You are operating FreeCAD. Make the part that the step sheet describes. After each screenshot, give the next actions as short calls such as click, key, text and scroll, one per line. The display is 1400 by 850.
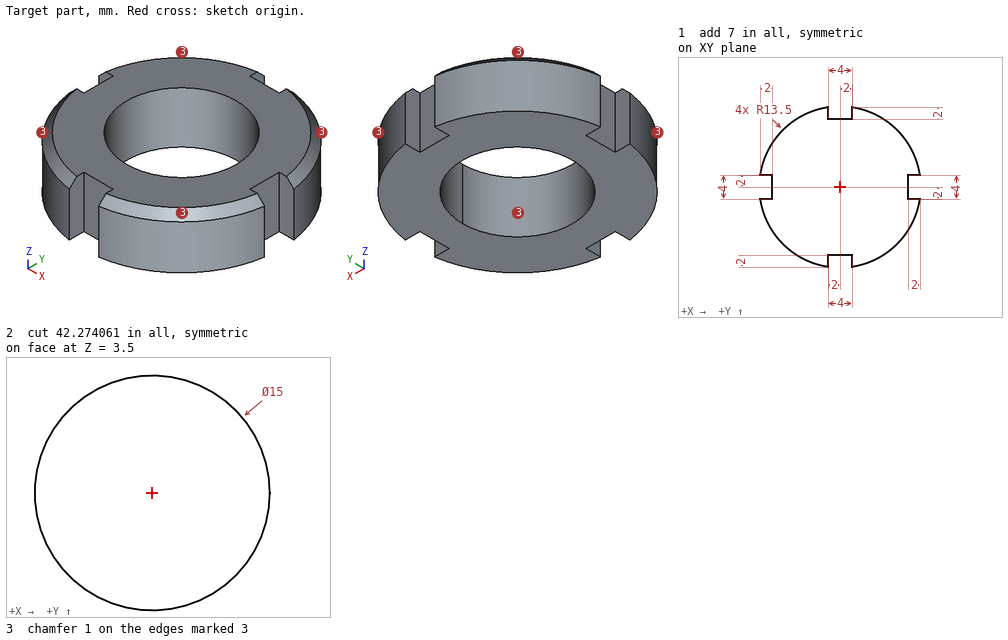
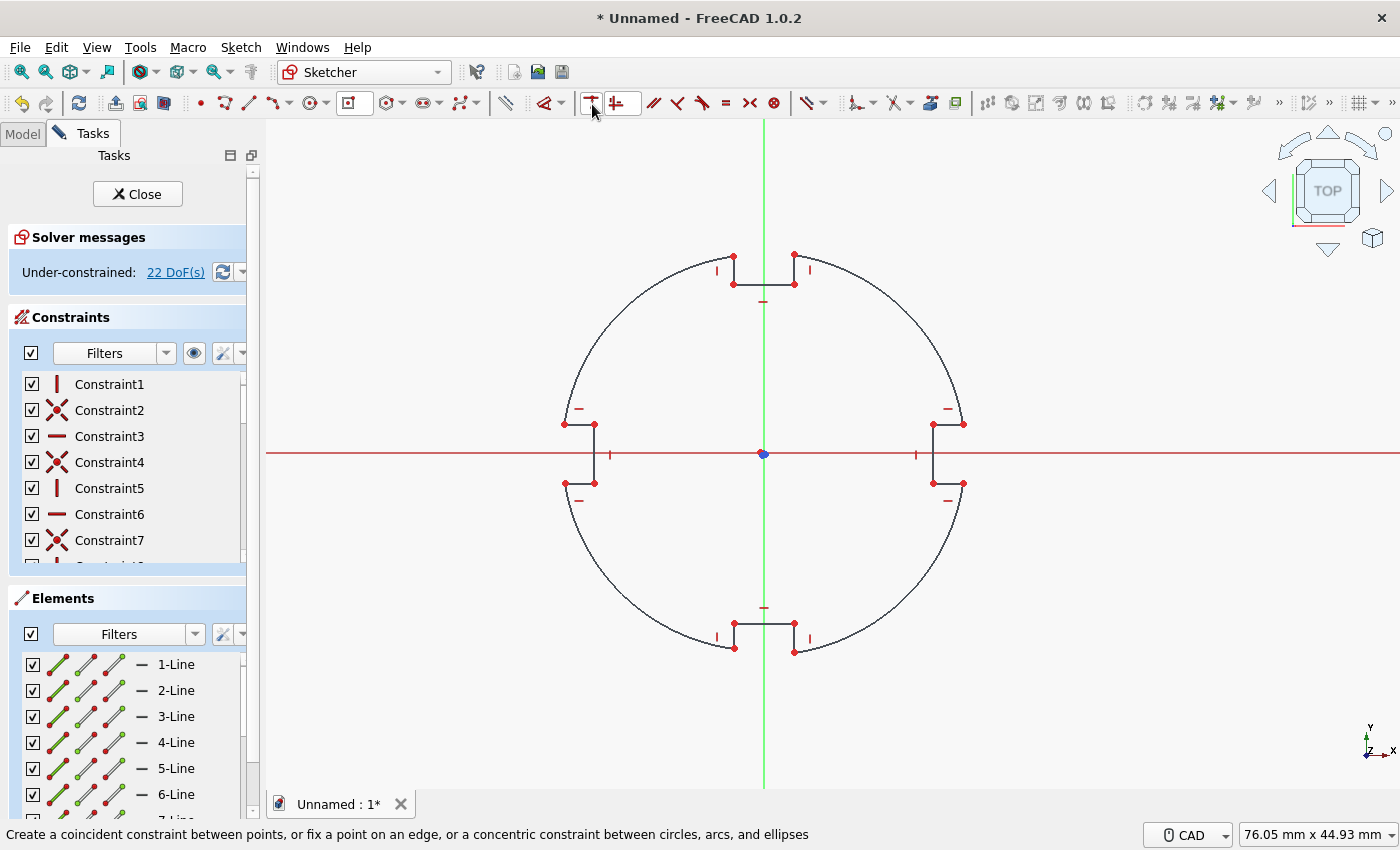
click(662, 281)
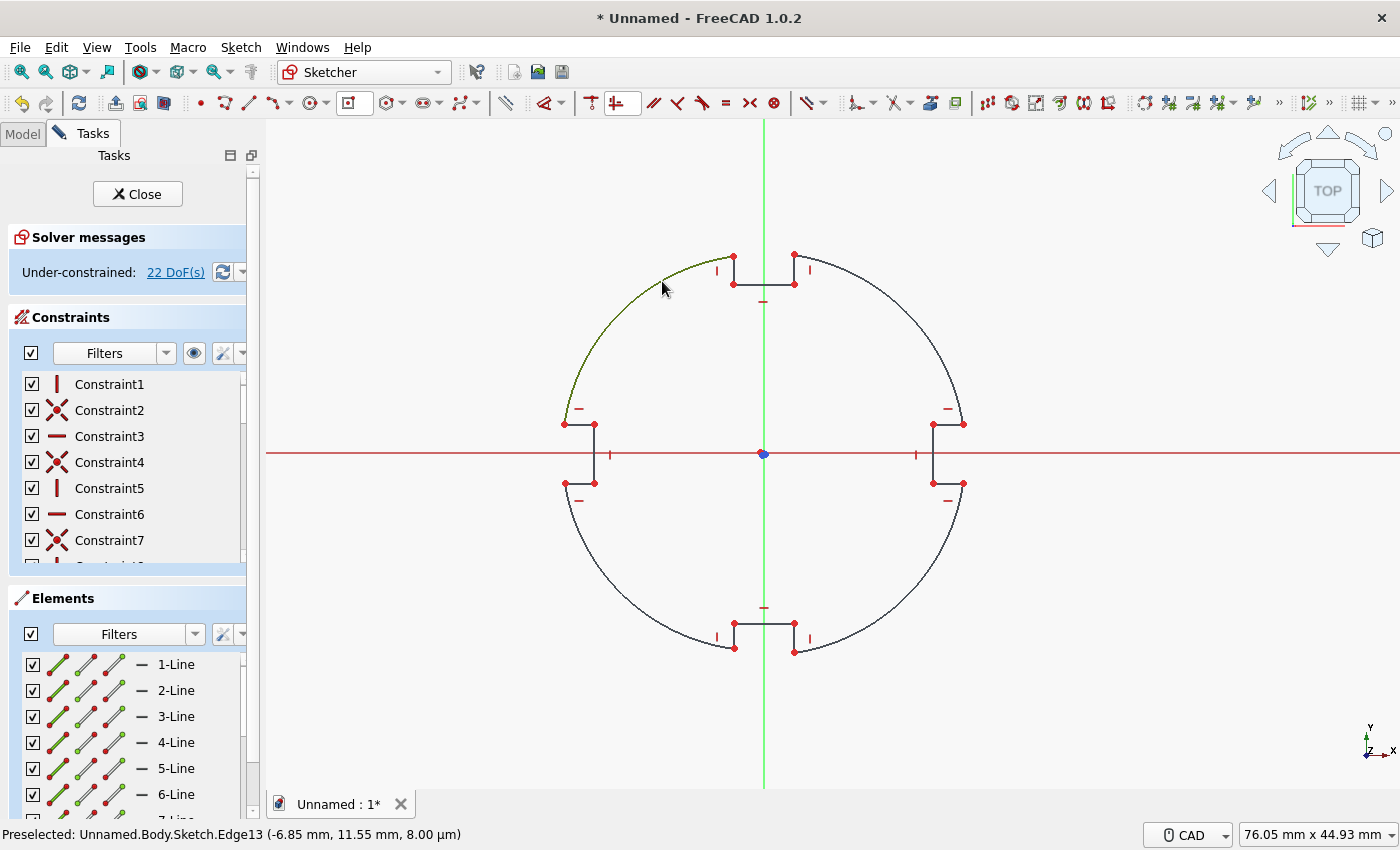
click(866, 628)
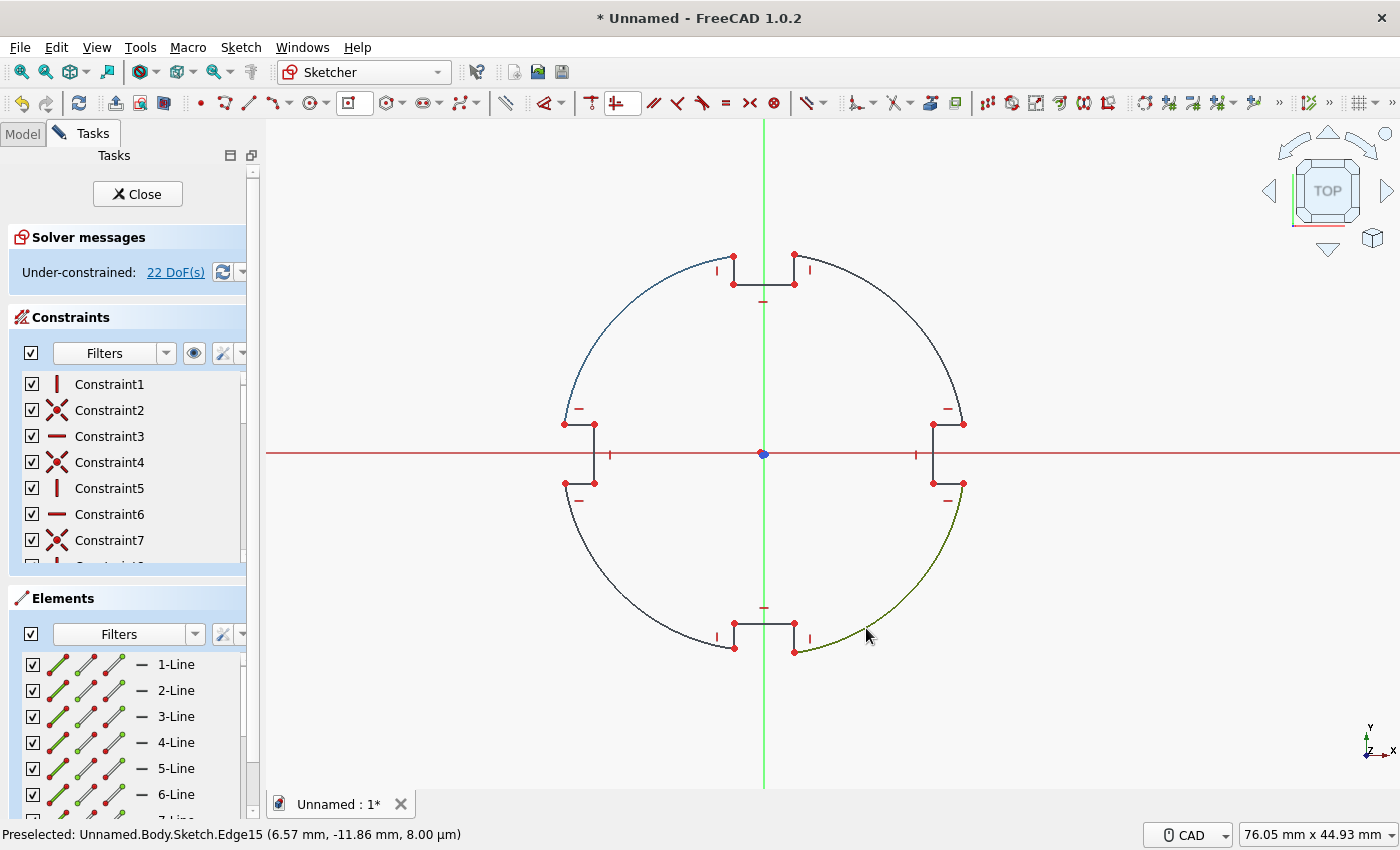
key(c)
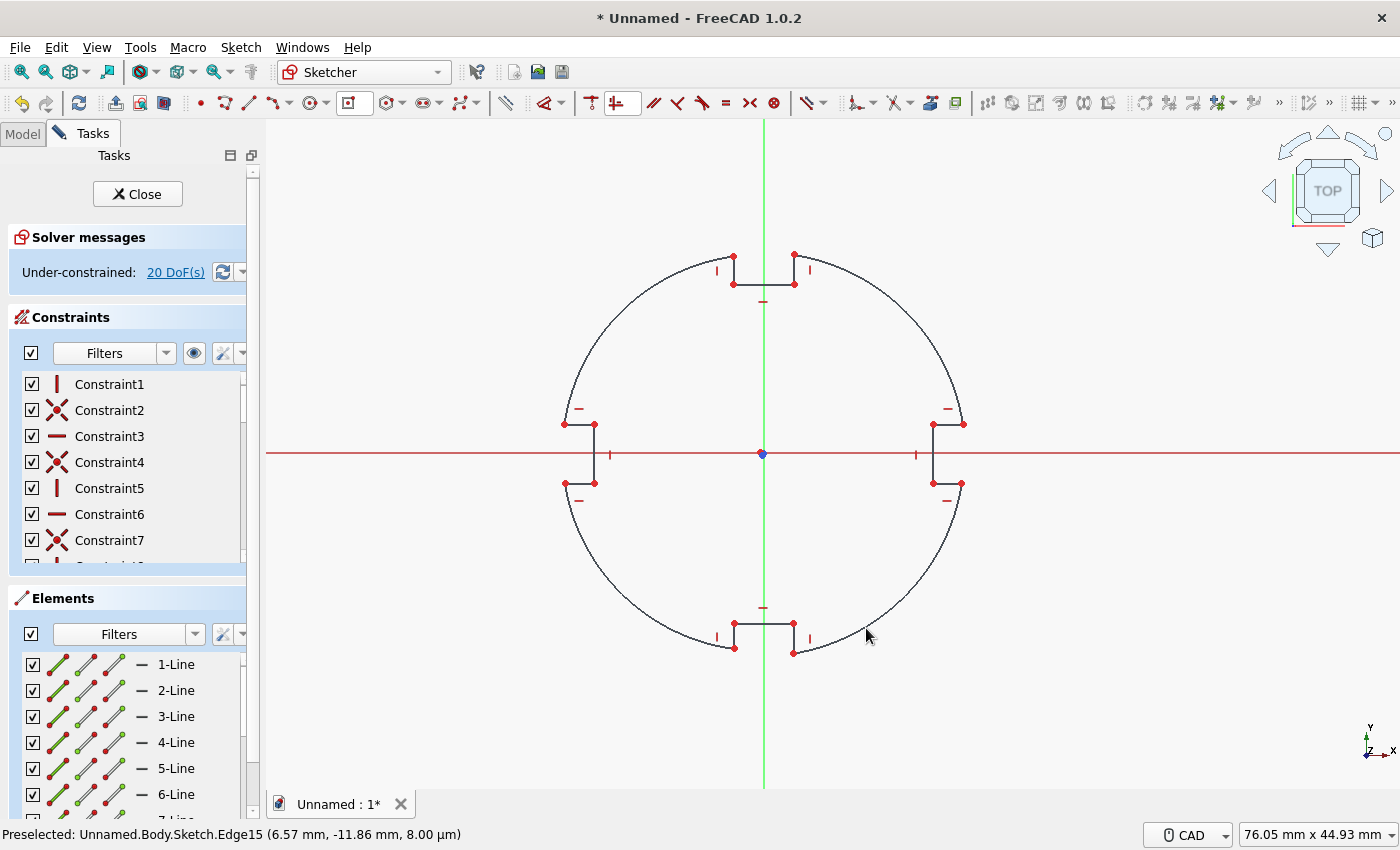
click(662, 281)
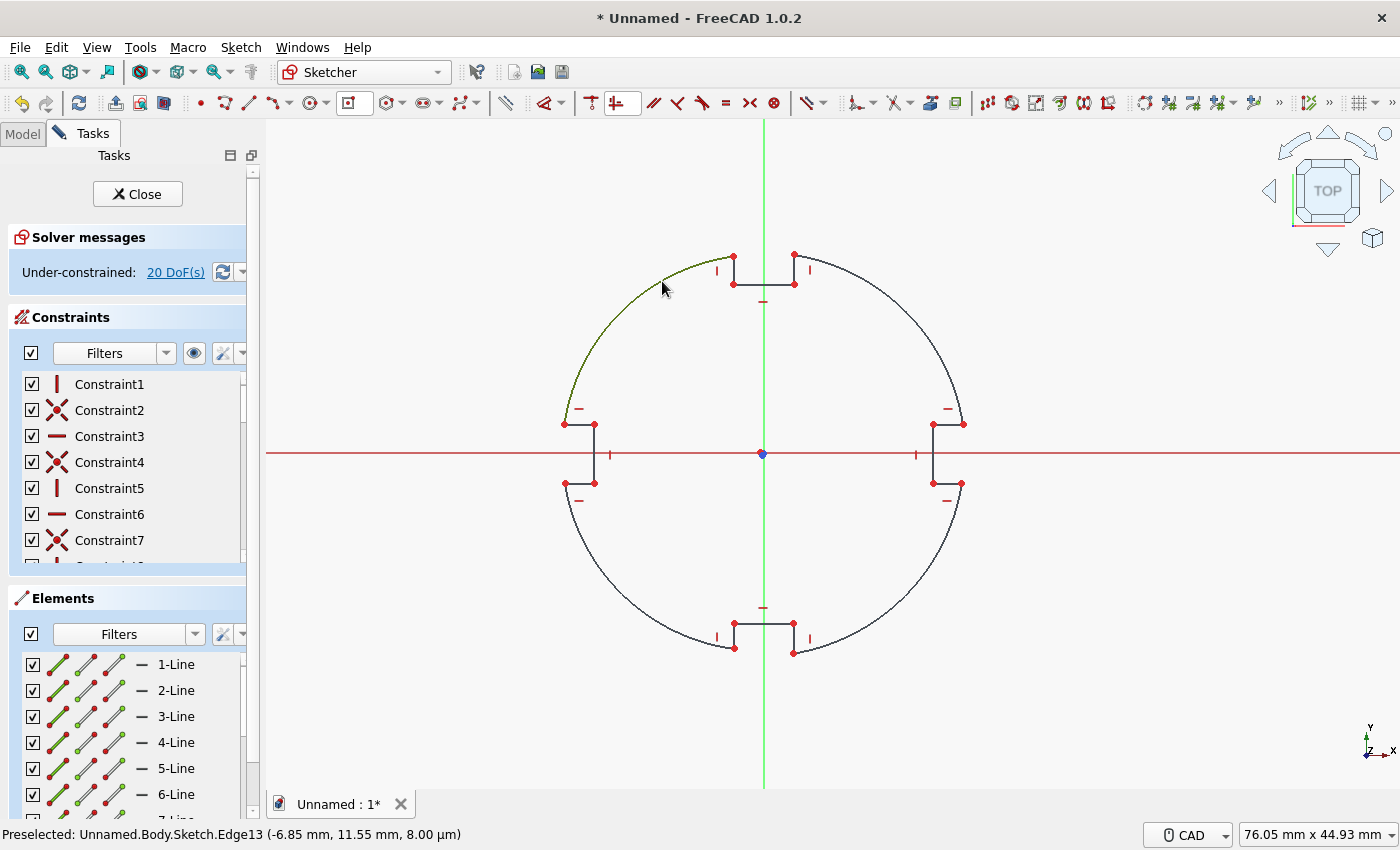
click(938, 353)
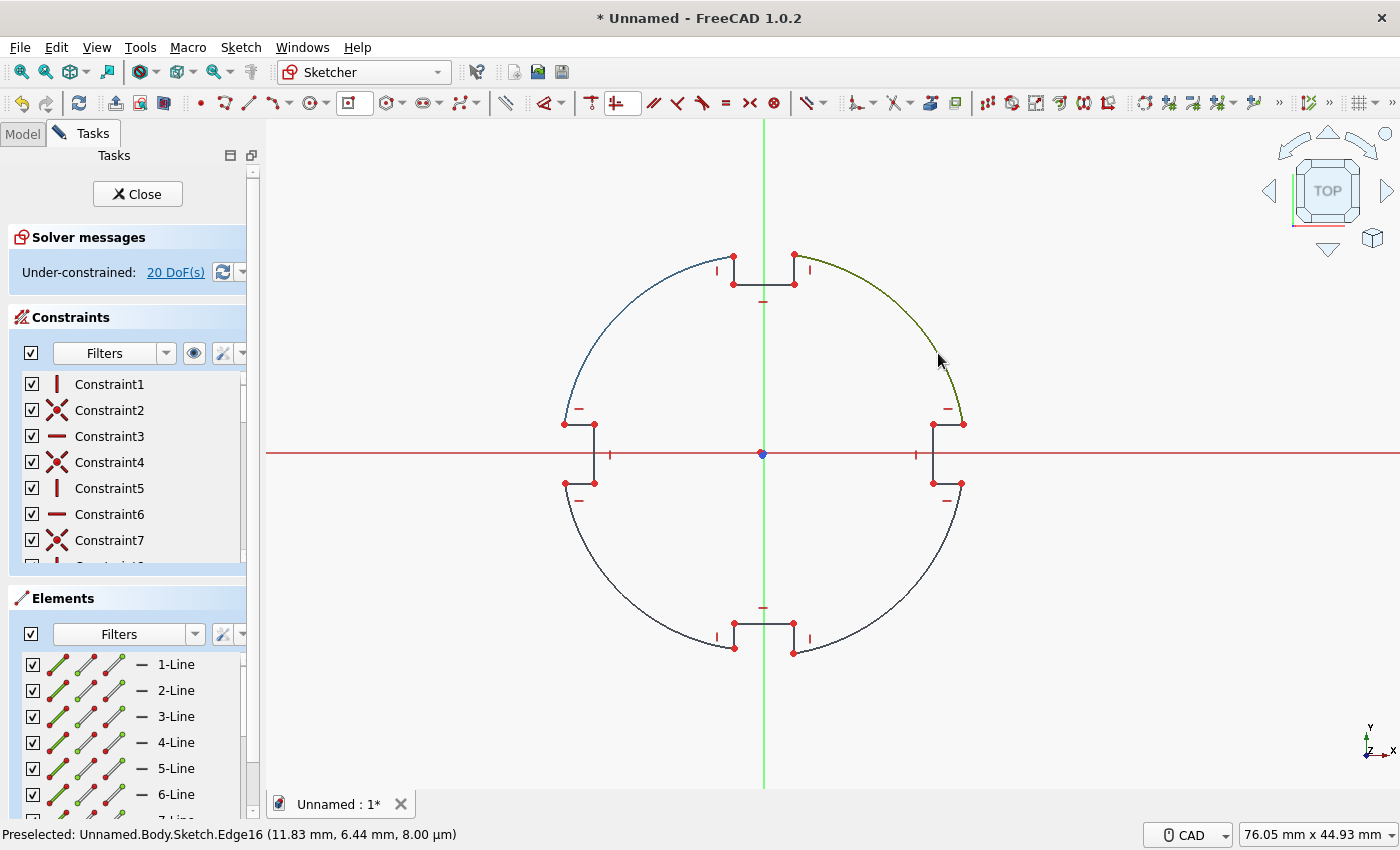
click(592, 104)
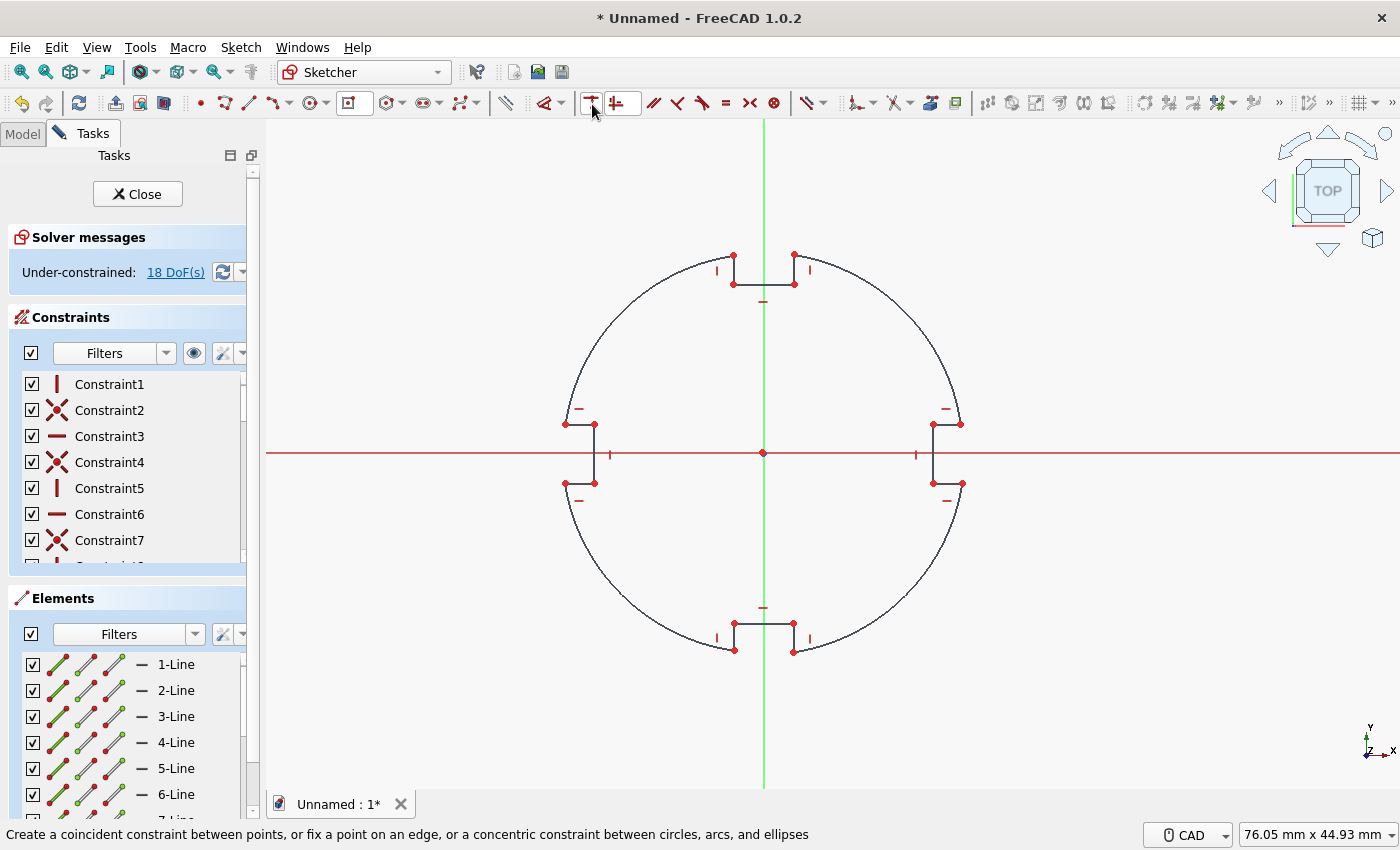
drag(753, 443, 774, 463)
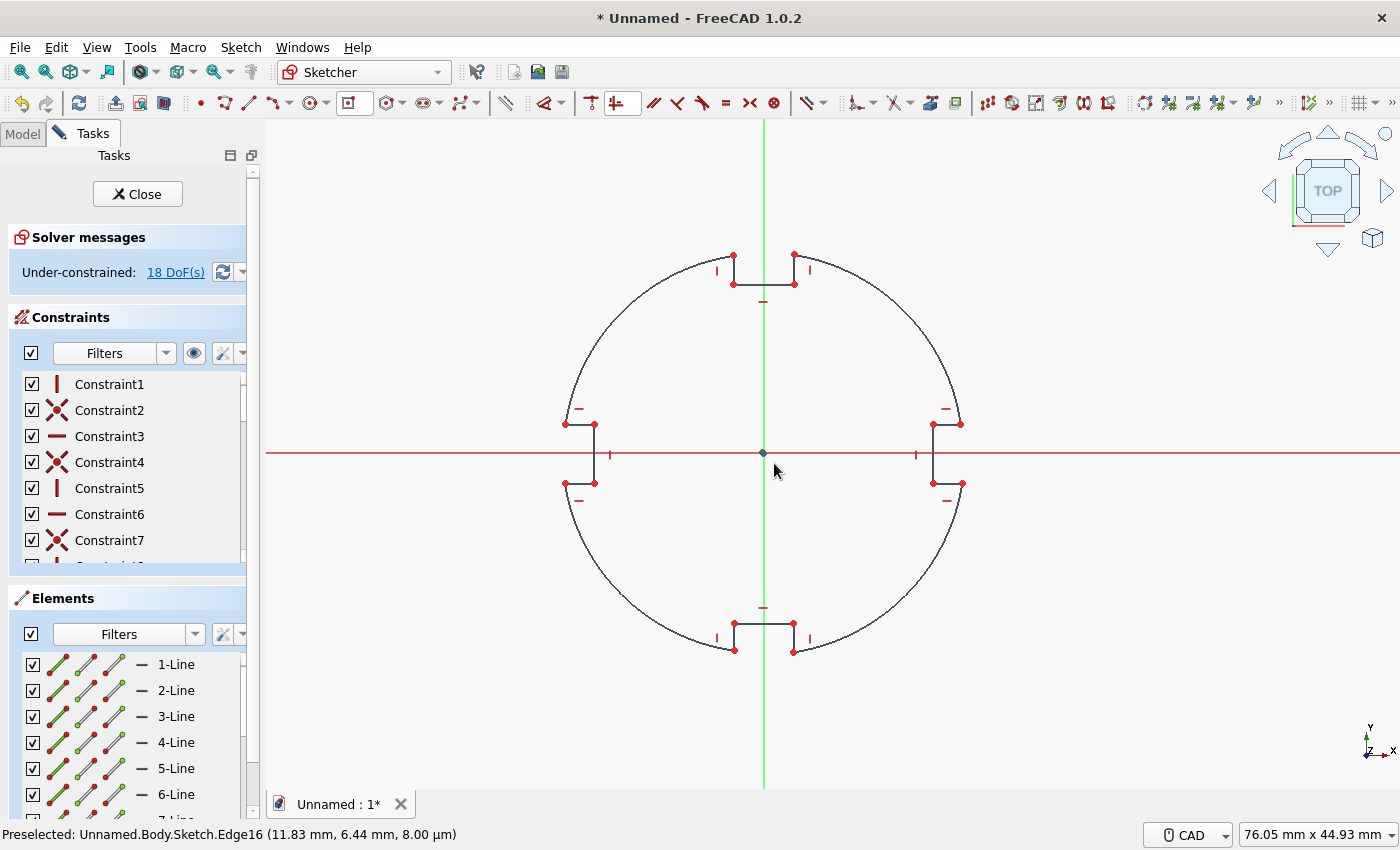
click(592, 104)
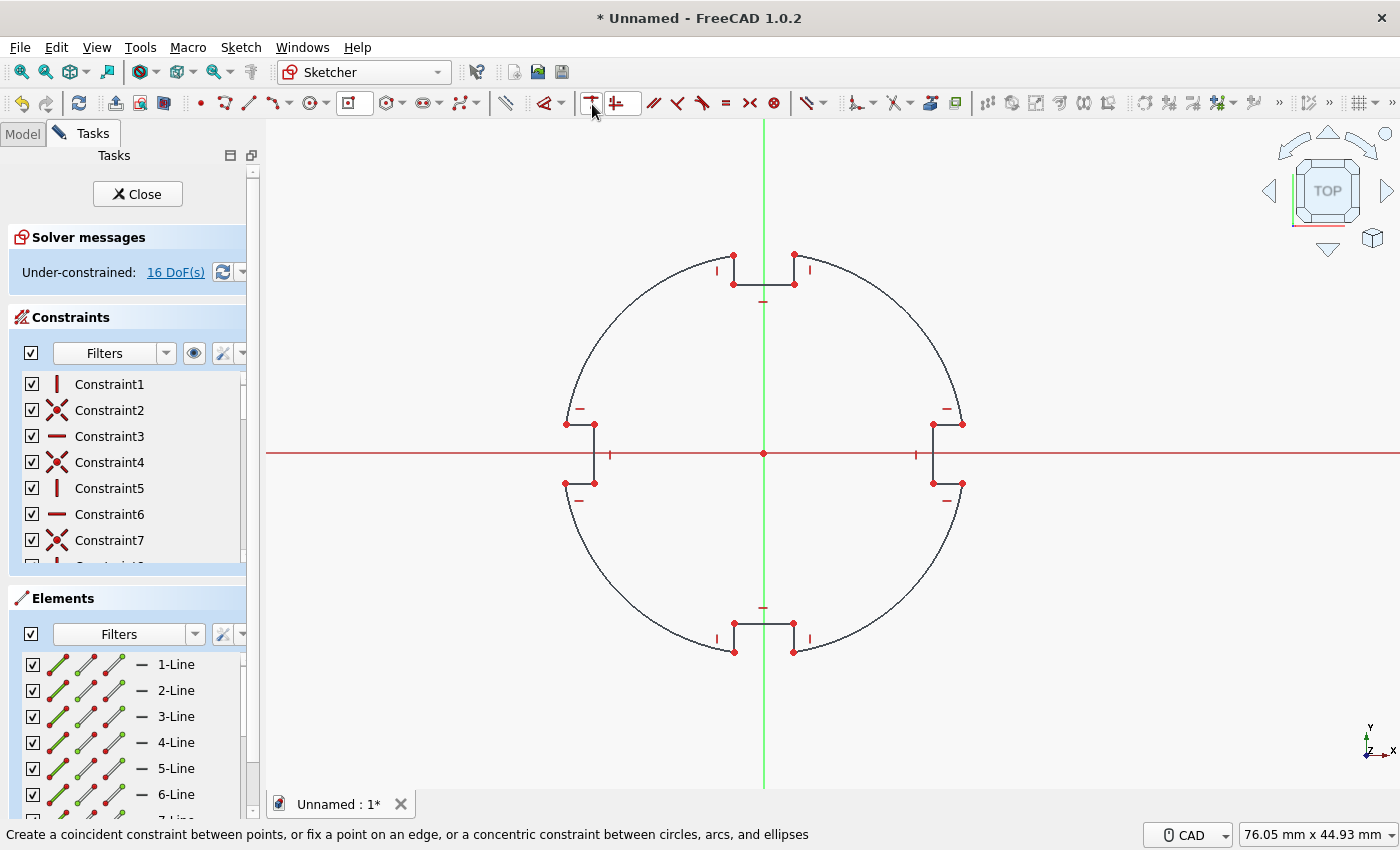
click(662, 281)